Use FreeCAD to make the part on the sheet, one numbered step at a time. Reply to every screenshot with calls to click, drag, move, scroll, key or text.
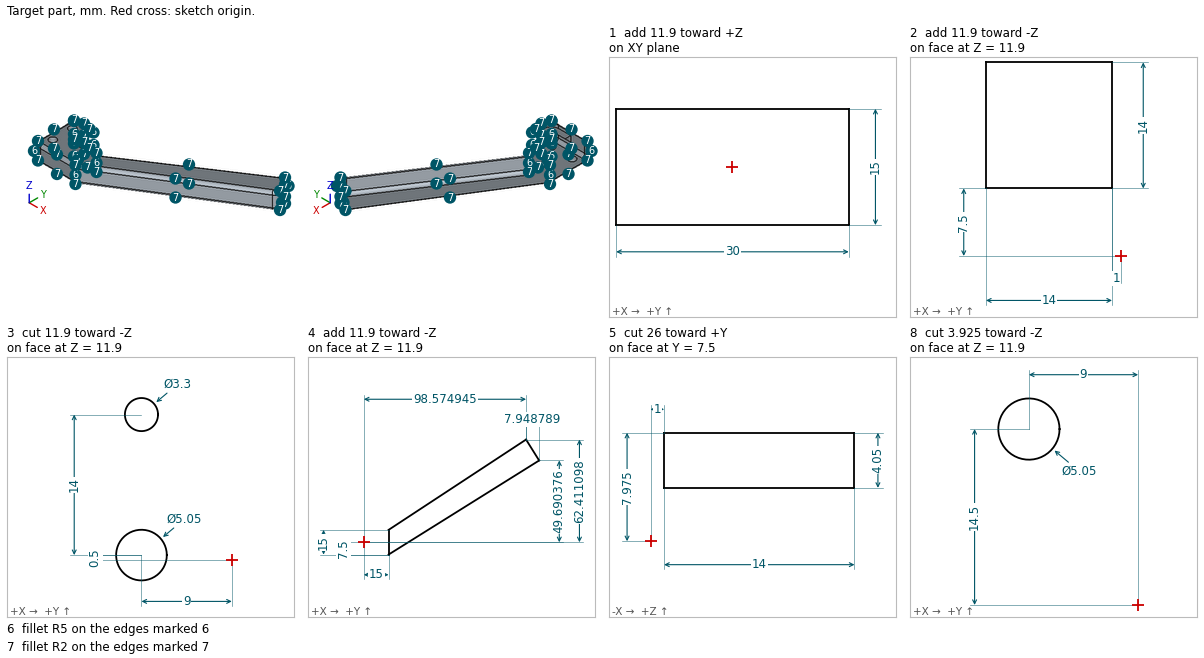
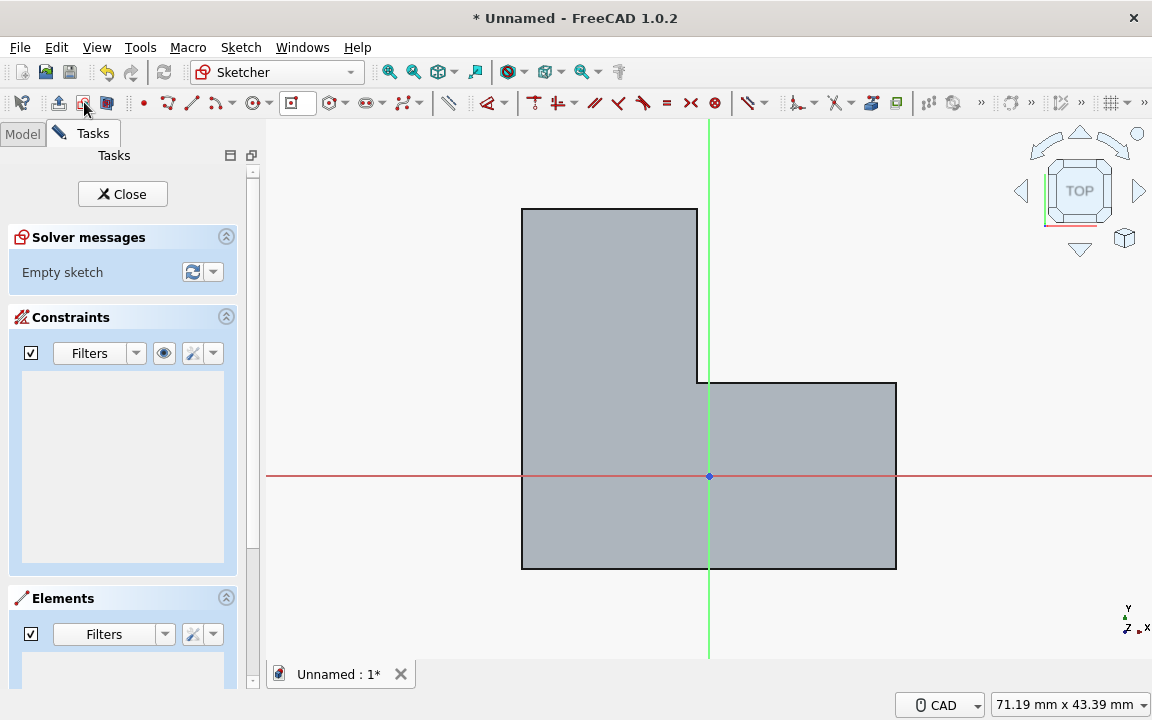
scroll(631, 387, up, 2)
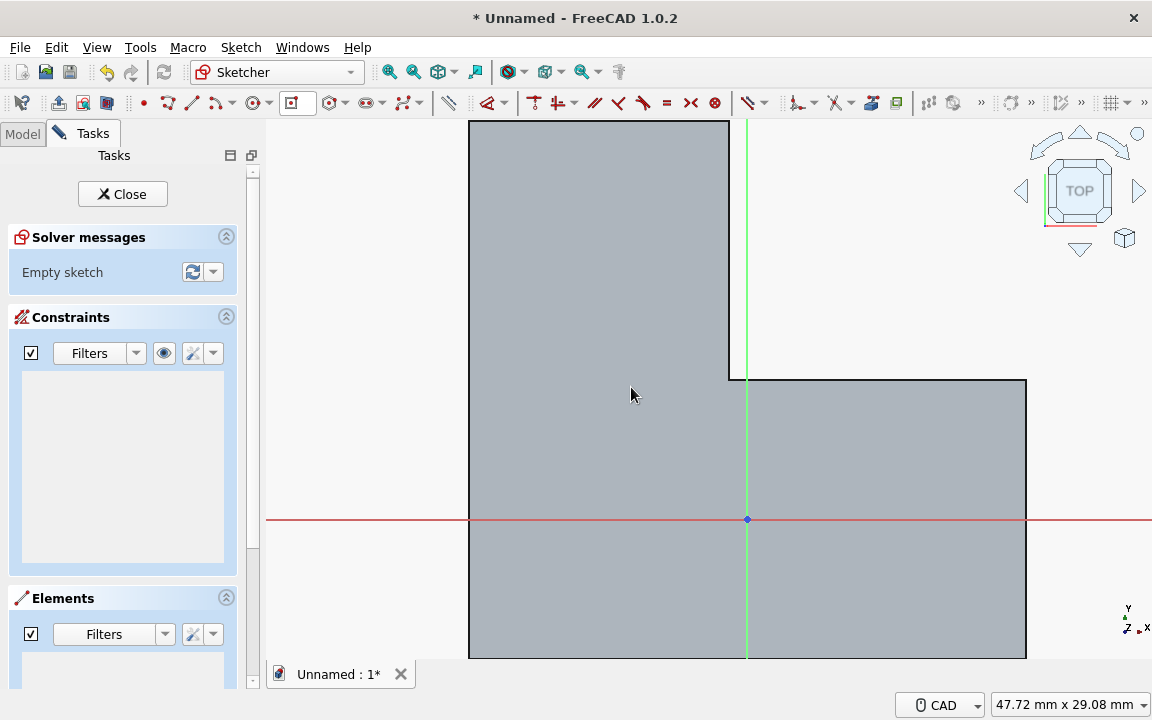
click(254, 104)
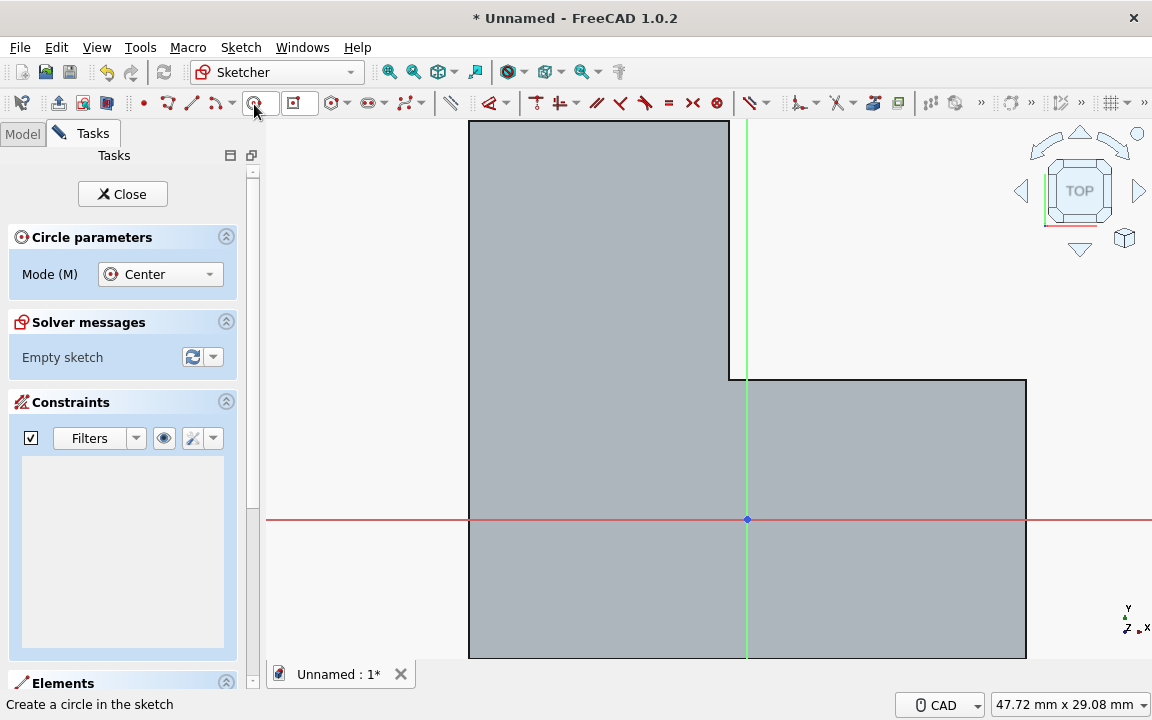
scroll(580, 510, up, 3)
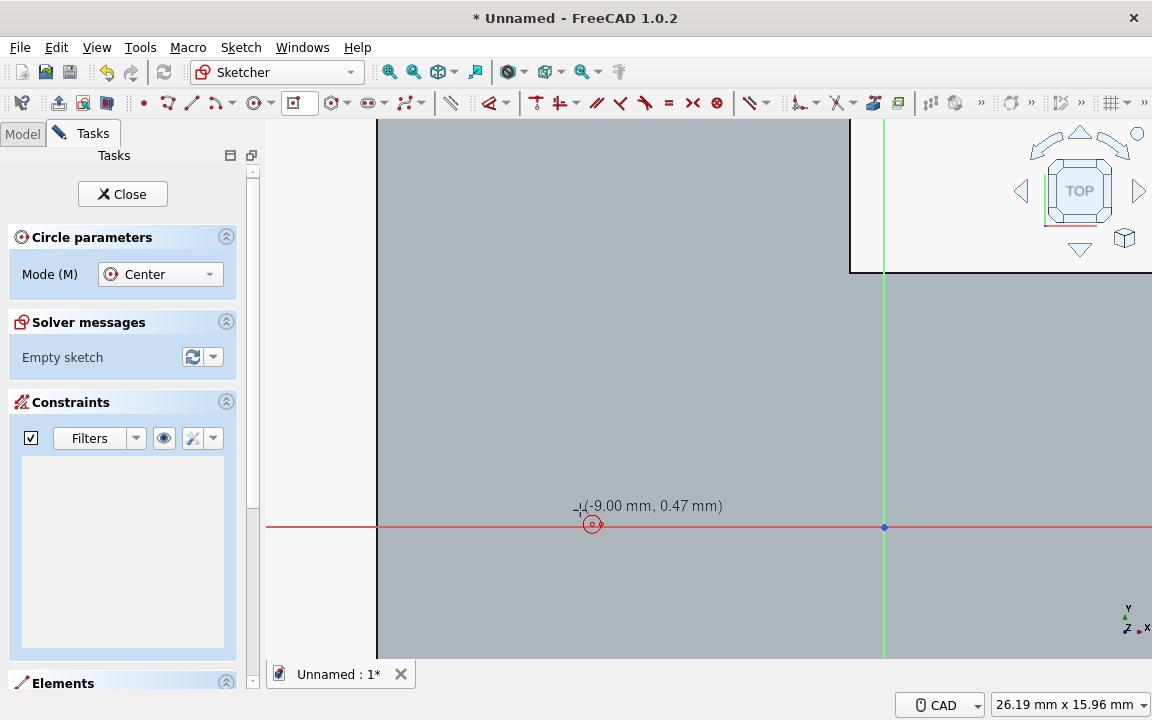
click(580, 510)
move(640, 450)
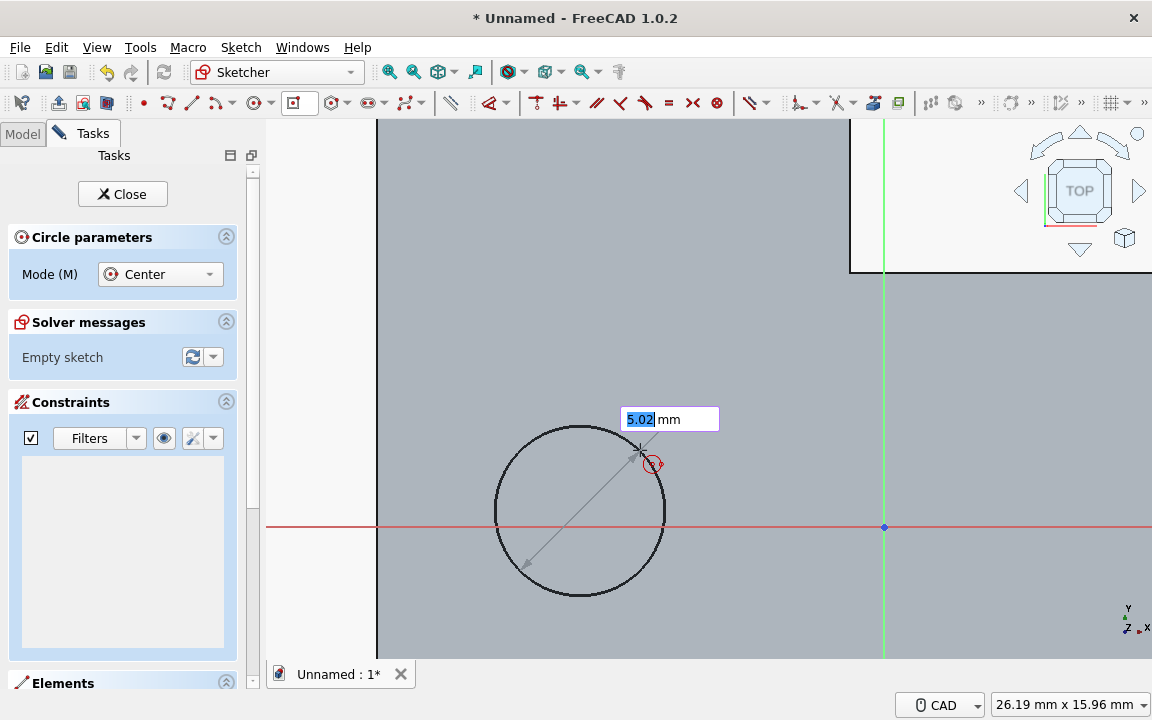
text(5.05)
key(Return)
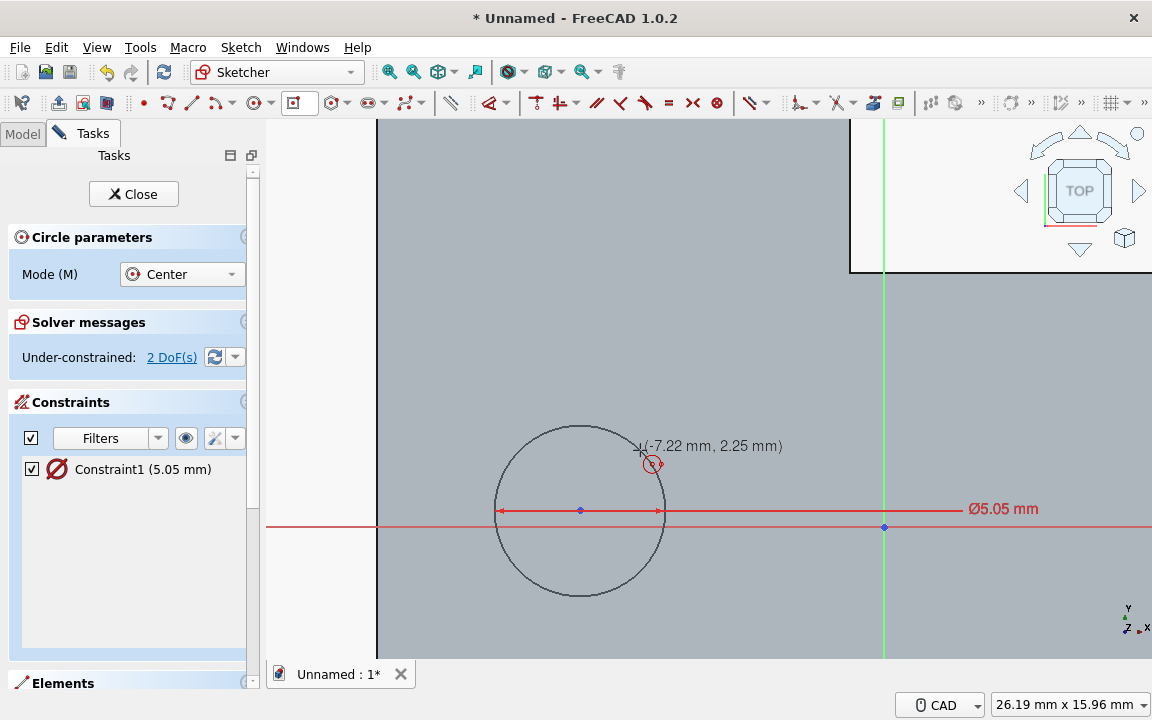
scroll(581, 512, down, 3)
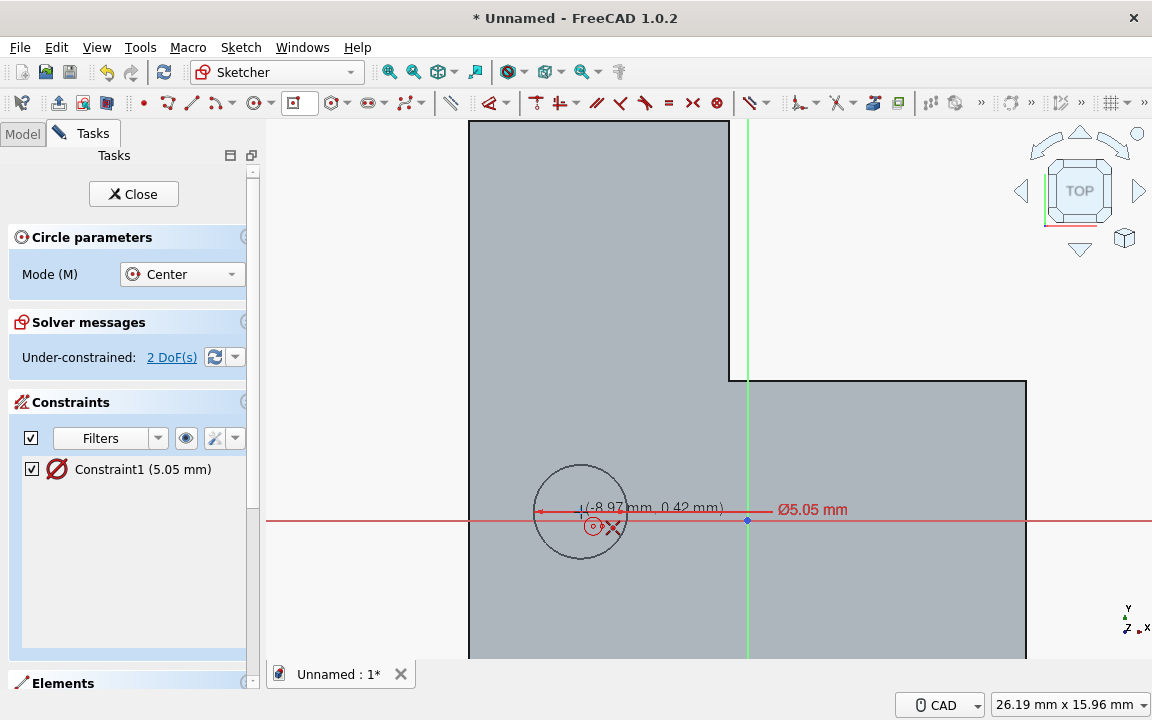
click(581, 251)
move(602, 230)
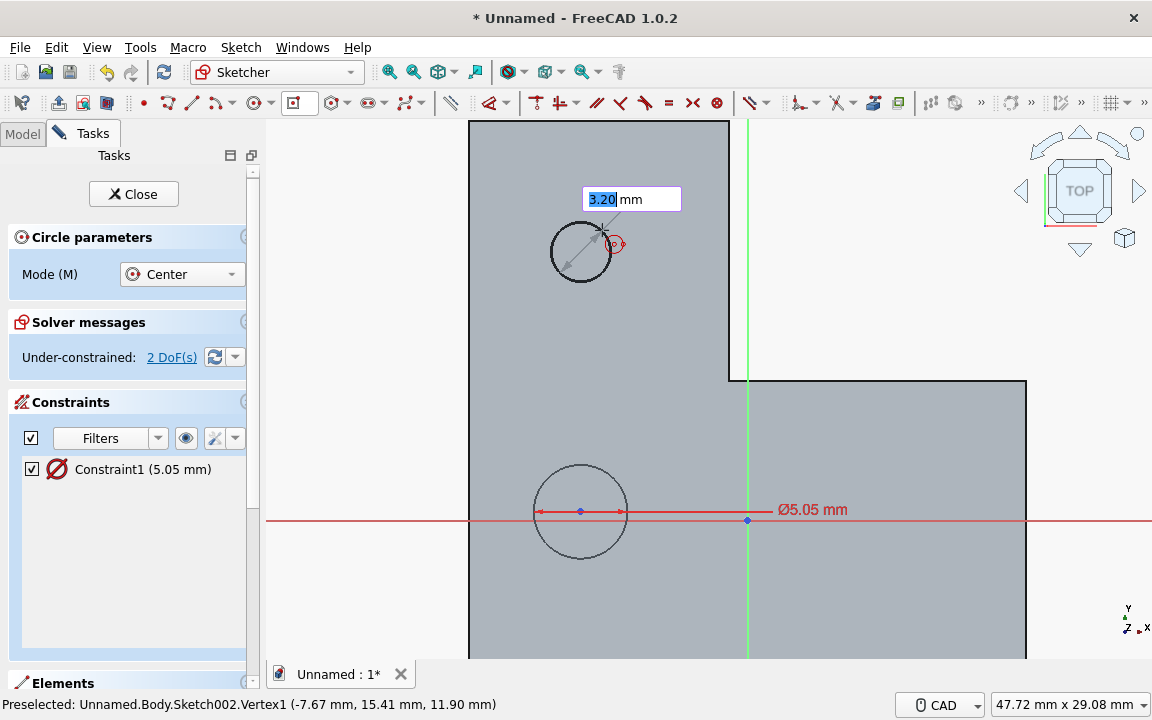
text(3.3)
key(Return)
key(Escape)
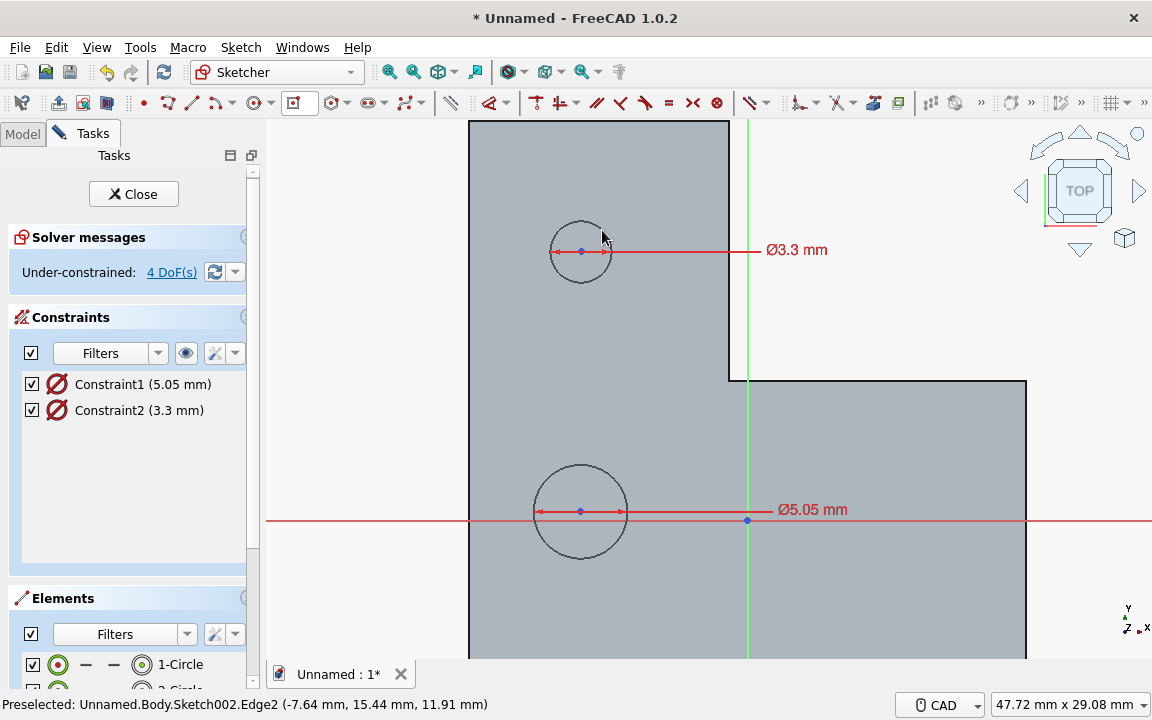
click(581, 512)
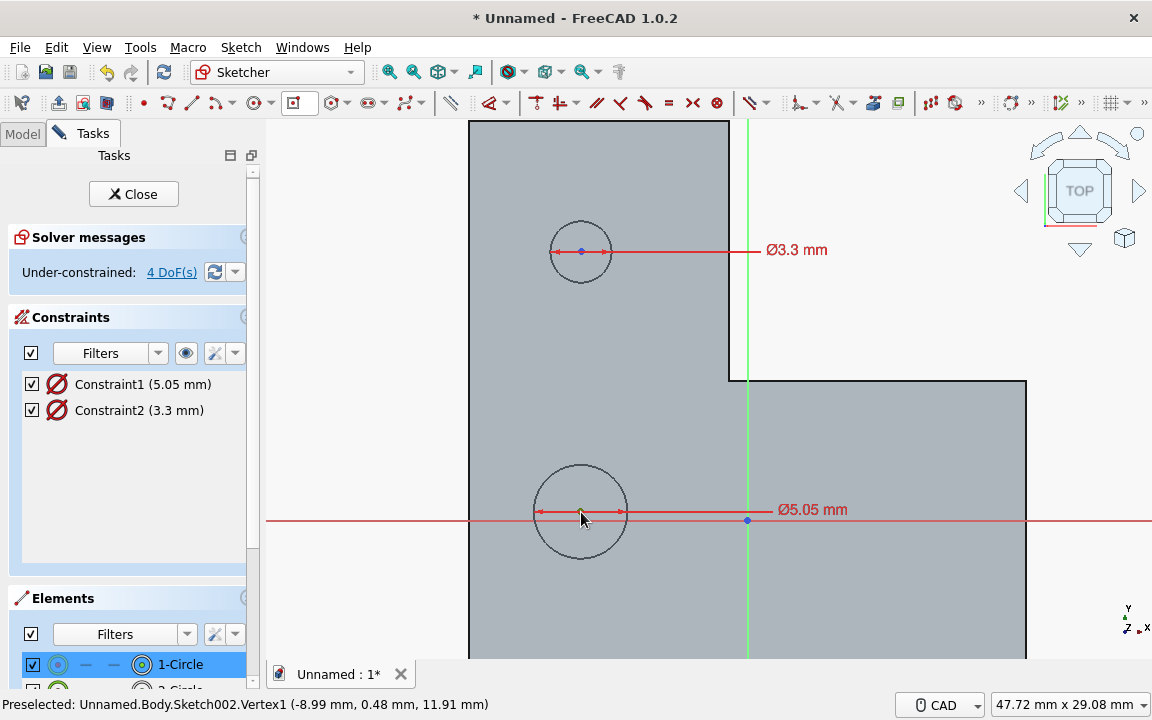
click(581, 252)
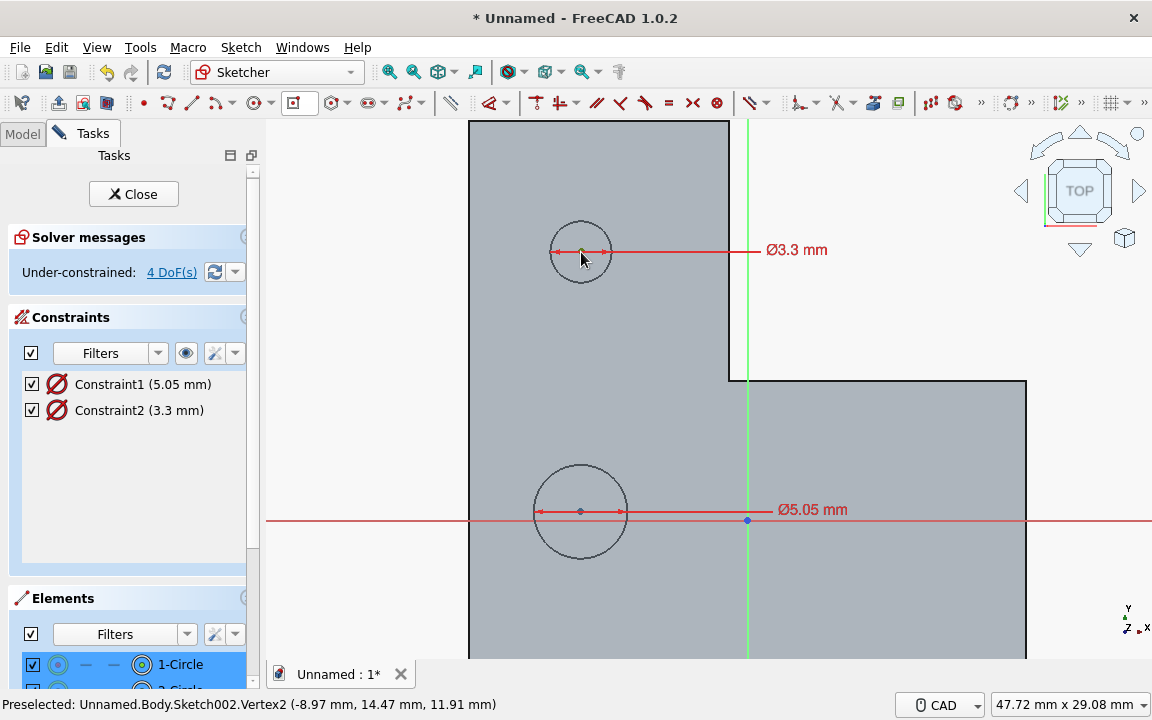
click(578, 104)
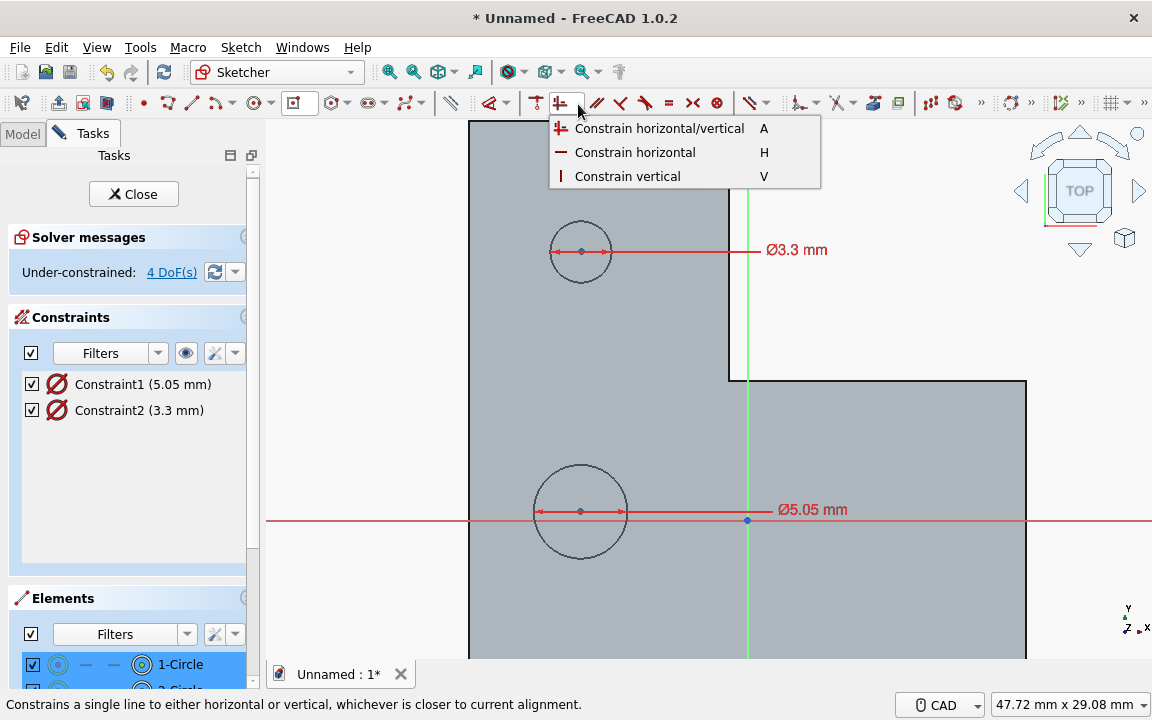
click(685, 176)